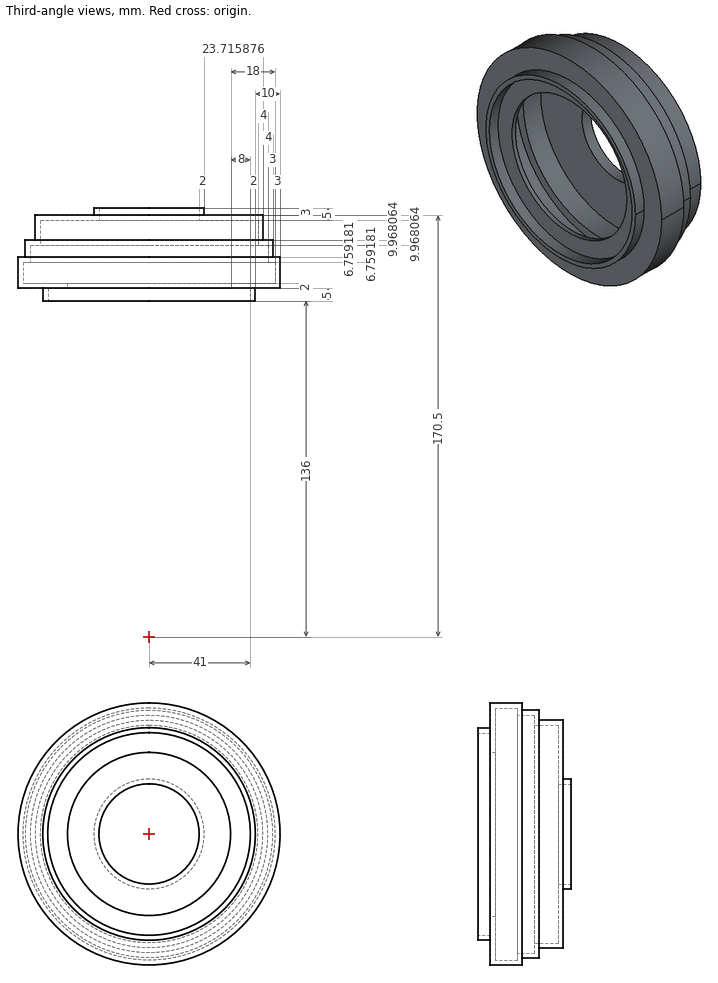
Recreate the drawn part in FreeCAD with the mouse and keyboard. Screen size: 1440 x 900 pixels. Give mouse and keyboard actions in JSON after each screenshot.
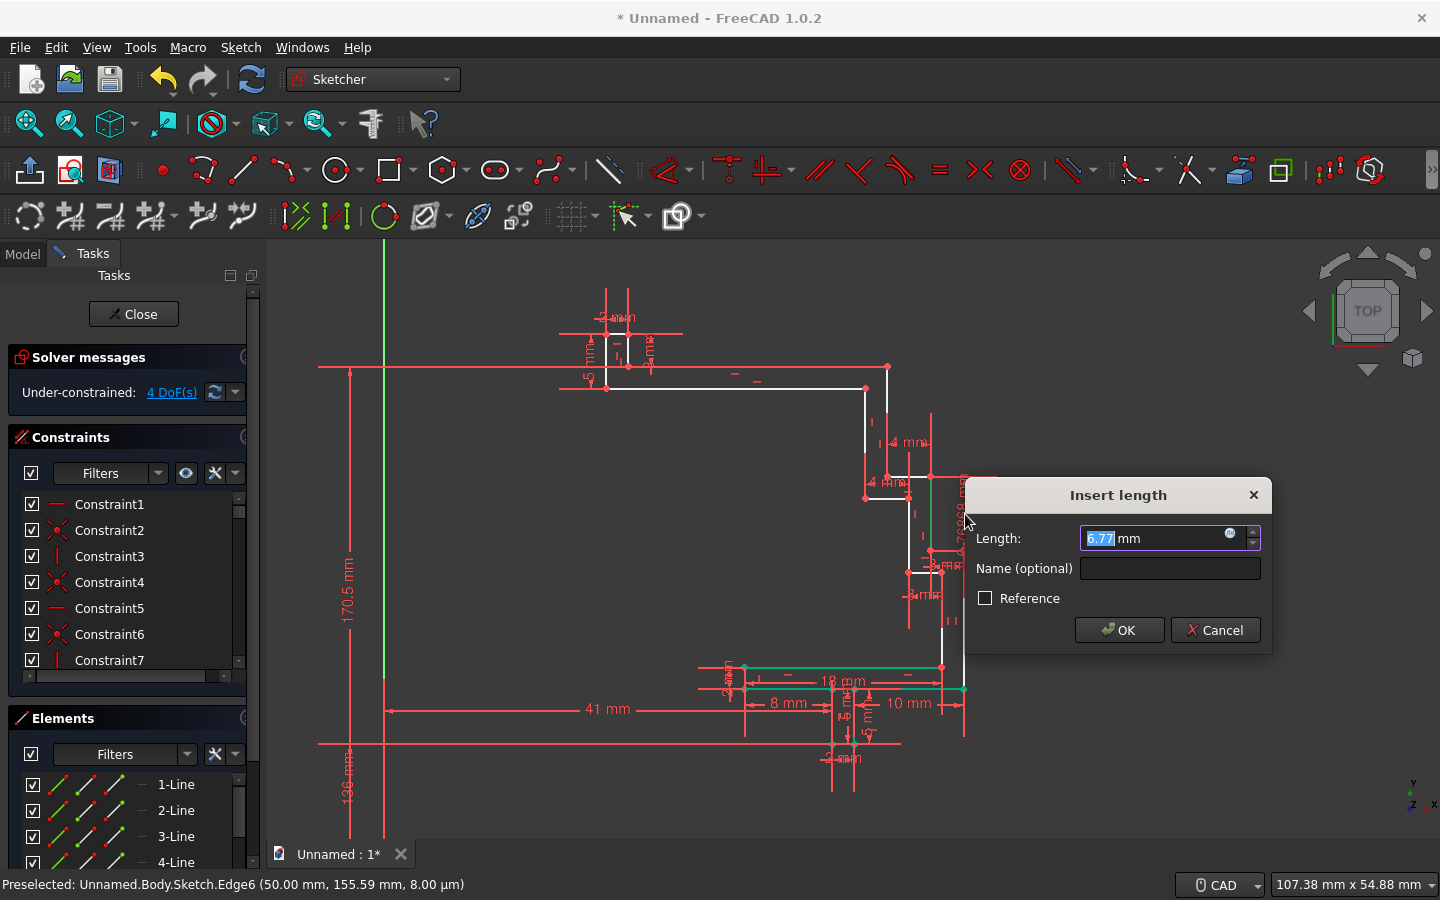
{"action": "type", "text": "6.759181"}
{"action": "key", "text": "Return"}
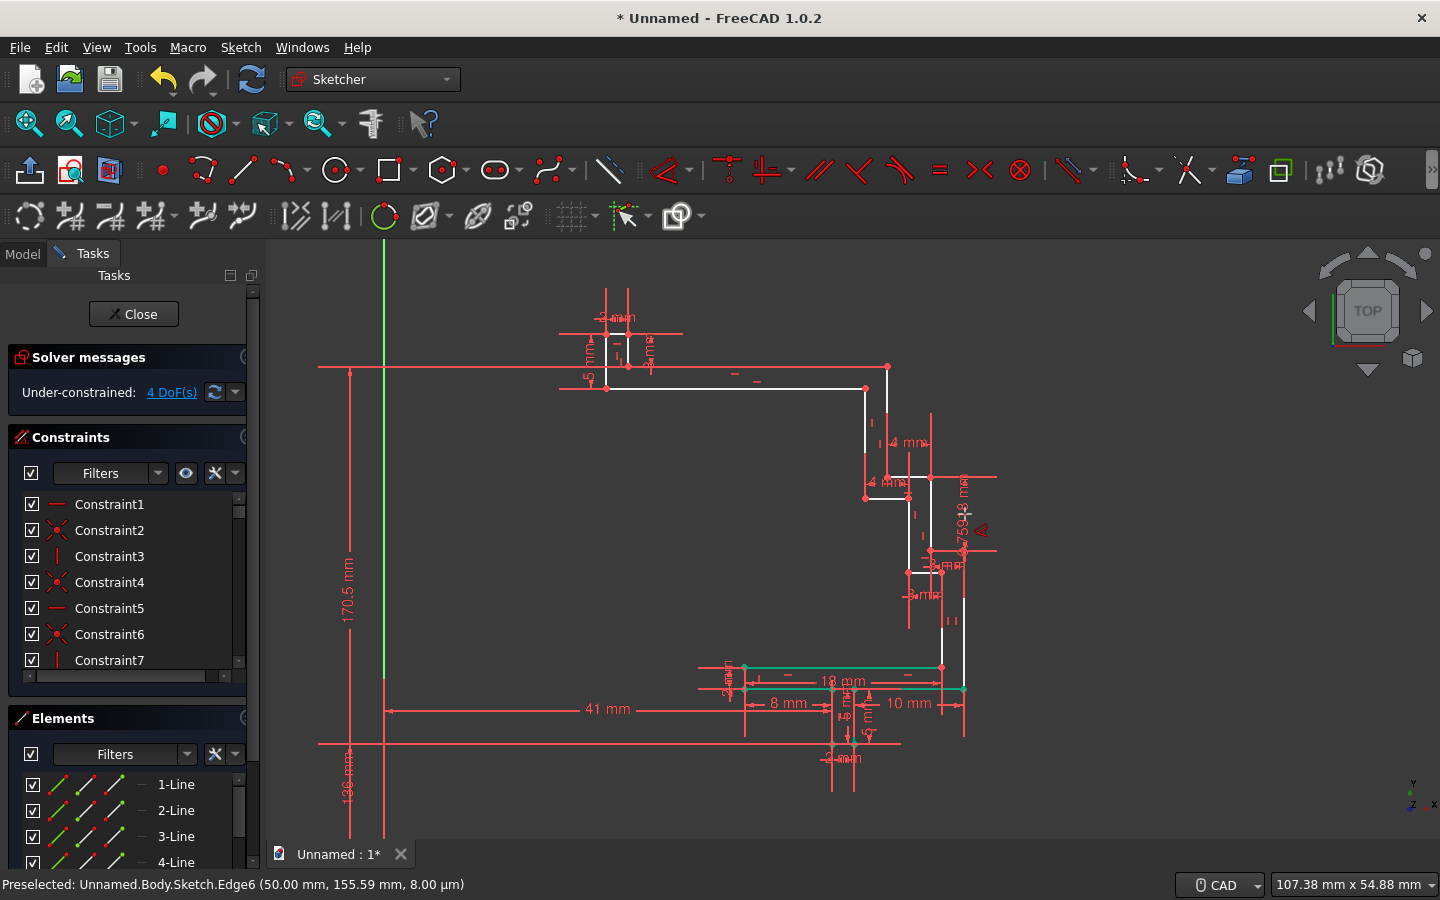
{"action": "left_click", "coordinate": [887, 444]}
{"action": "left_click", "coordinate": [921, 422]}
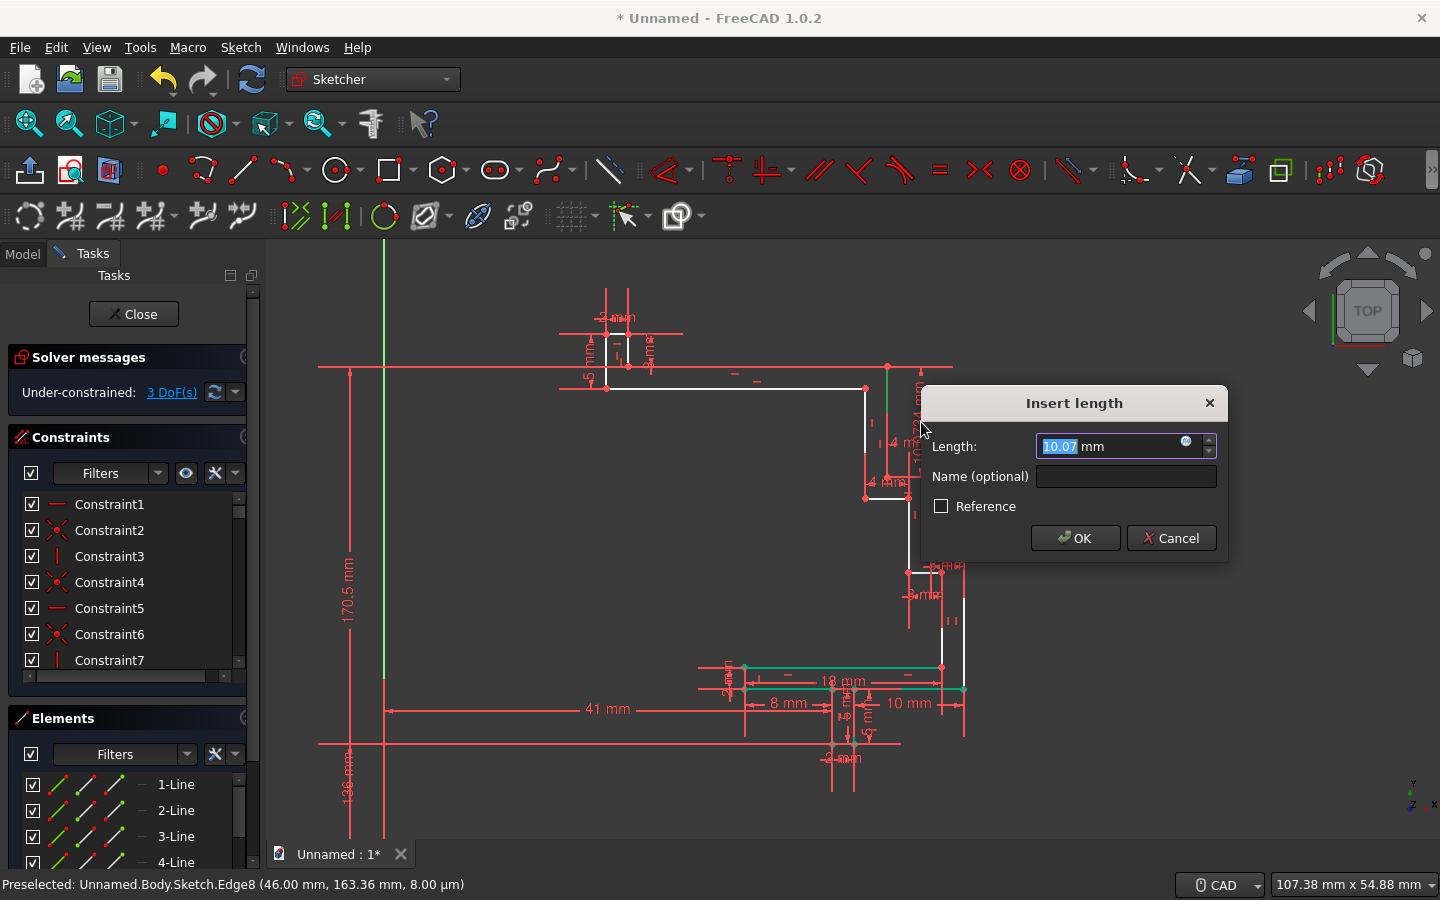
{"action": "type", "text": "9.968064"}
{"action": "key", "text": "Return"}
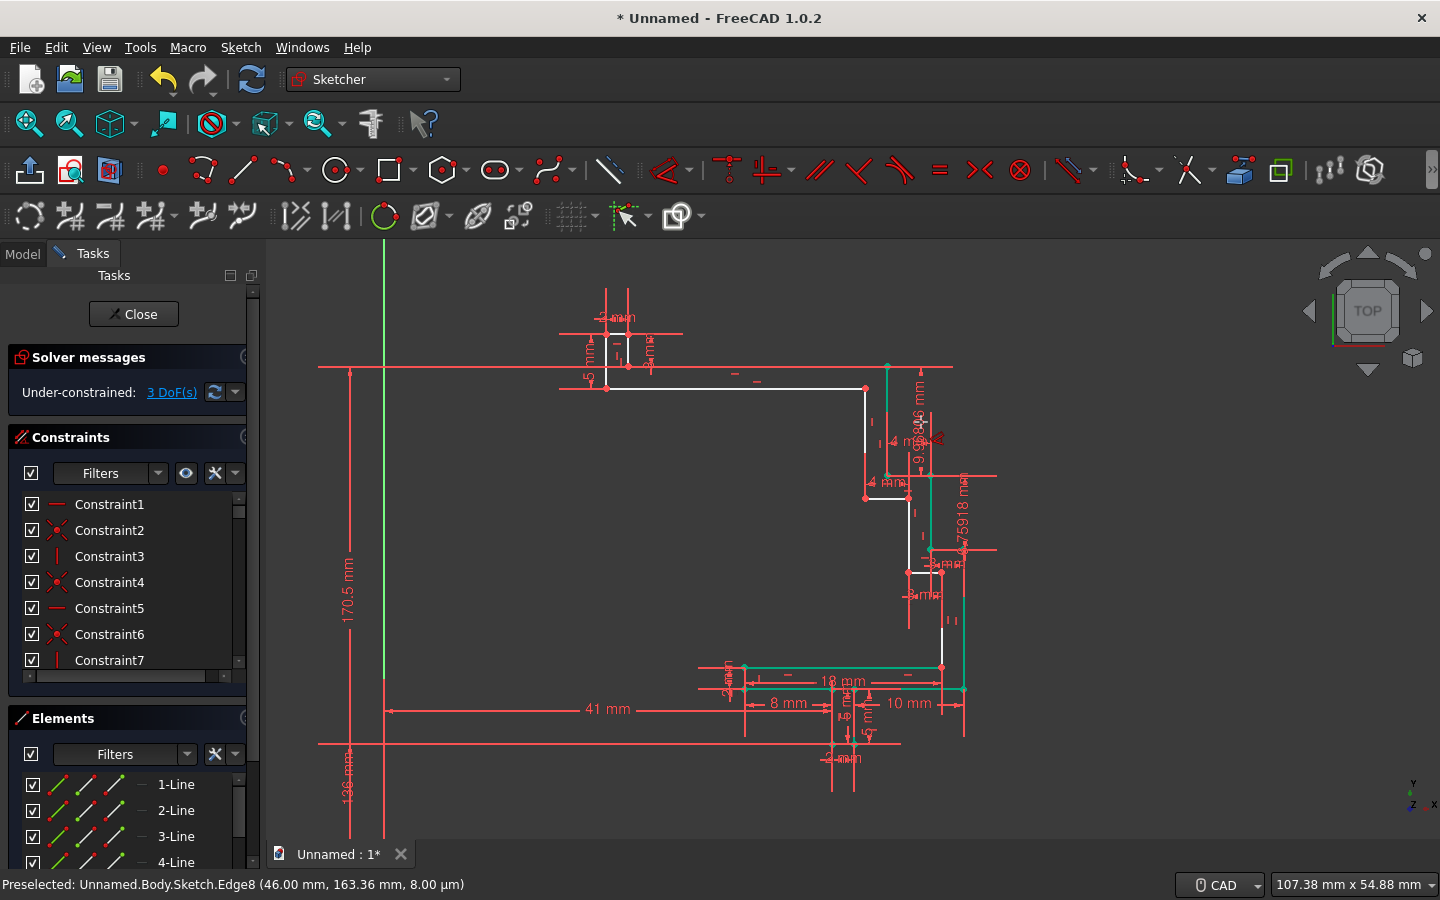
{"action": "left_click", "coordinate": [865, 422]}
{"action": "left_click", "coordinate": [831, 444]}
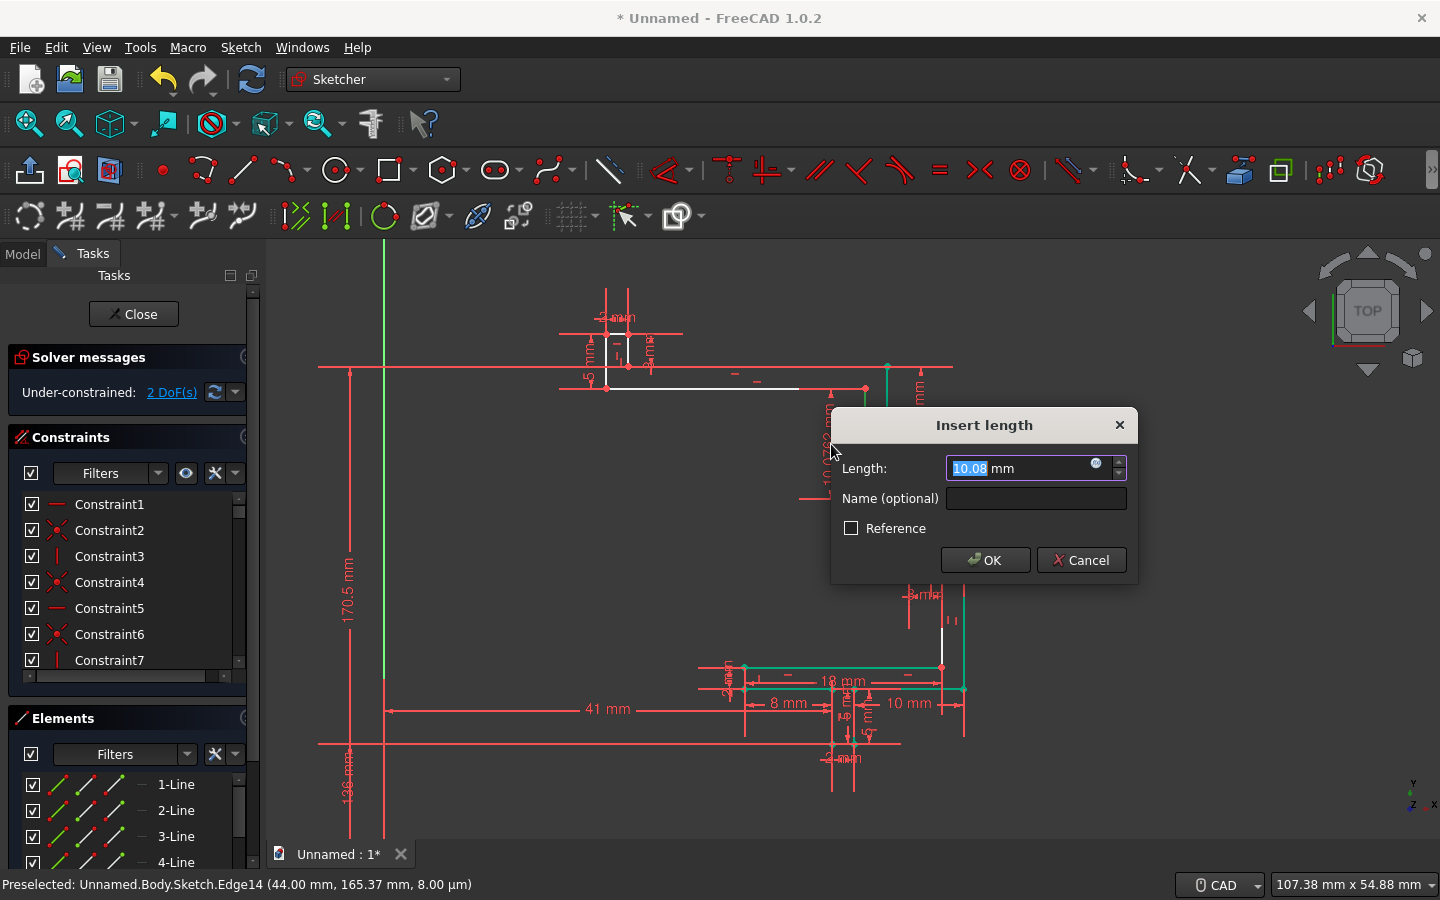
{"action": "type", "text": "9.968064"}
{"action": "key", "text": "Return"}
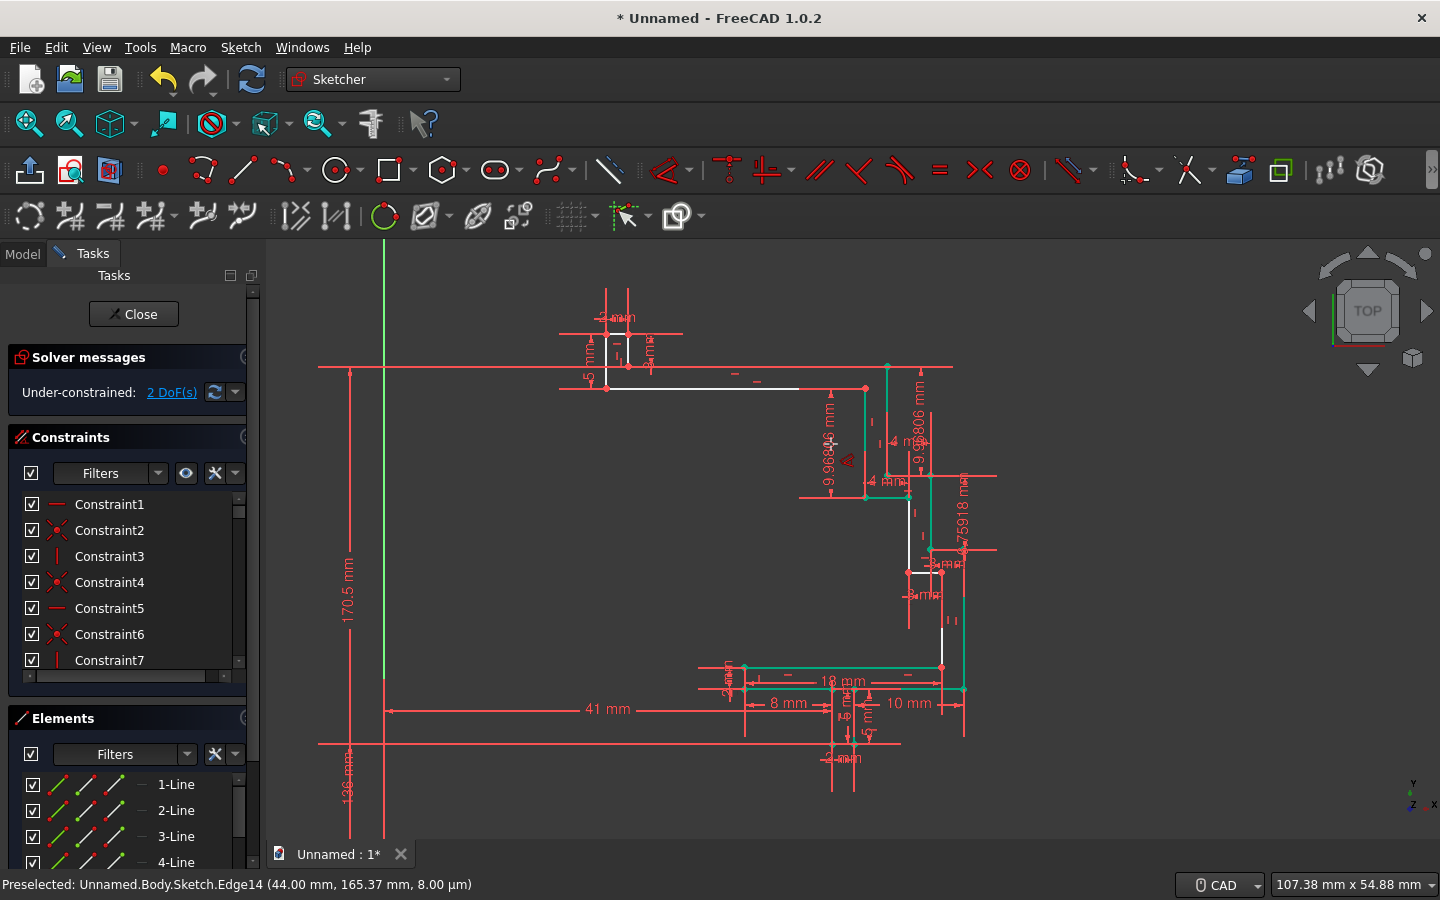
{"action": "left_click", "coordinate": [909, 520]}
{"action": "left_click", "coordinate": [875, 535]}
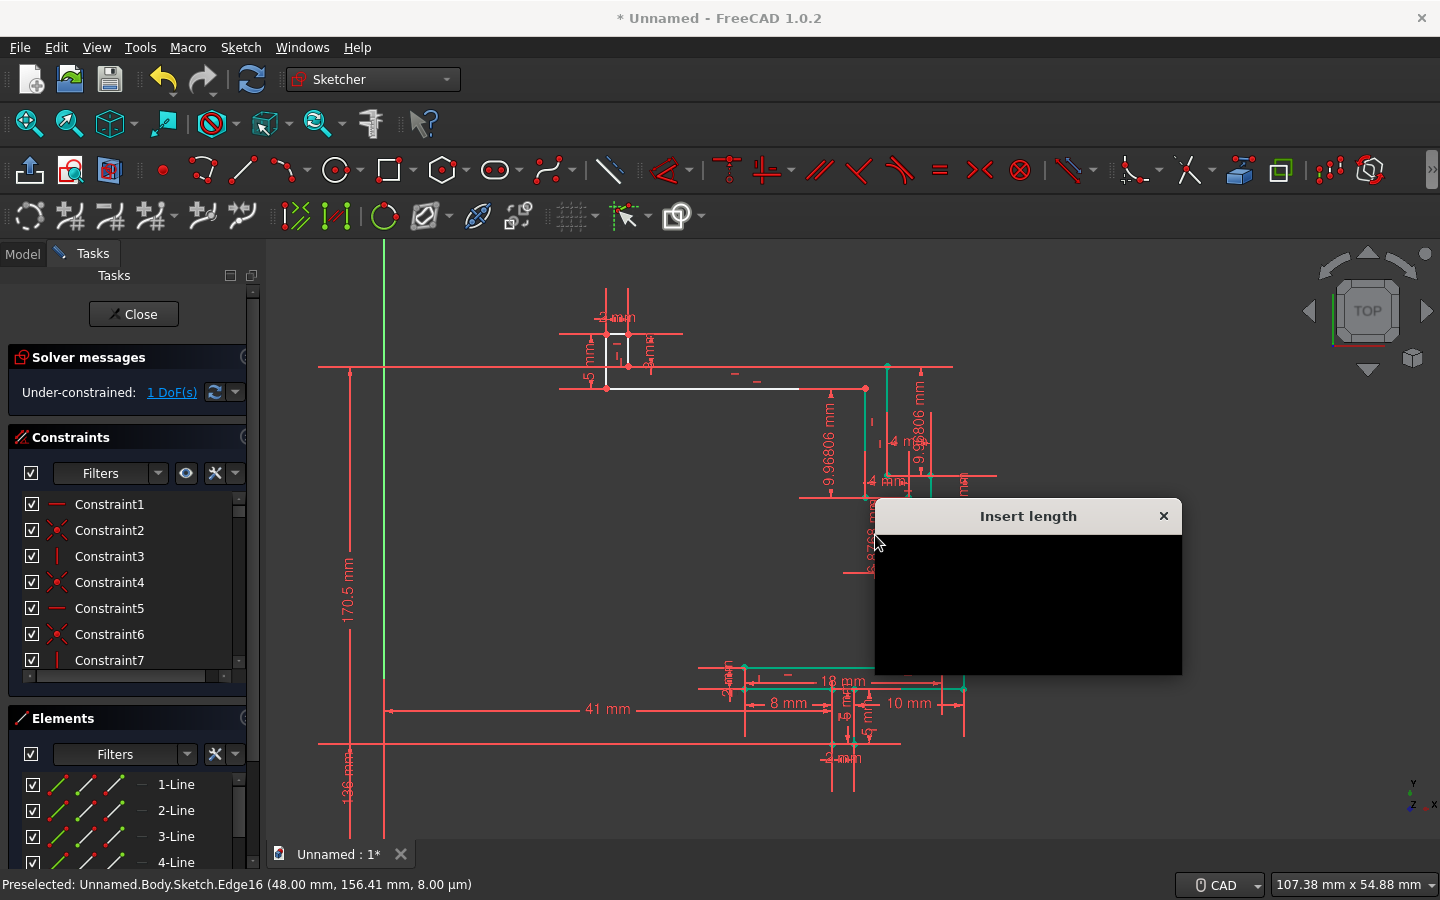
{"action": "type", "text": "6.759181"}
{"action": "key", "text": "Return"}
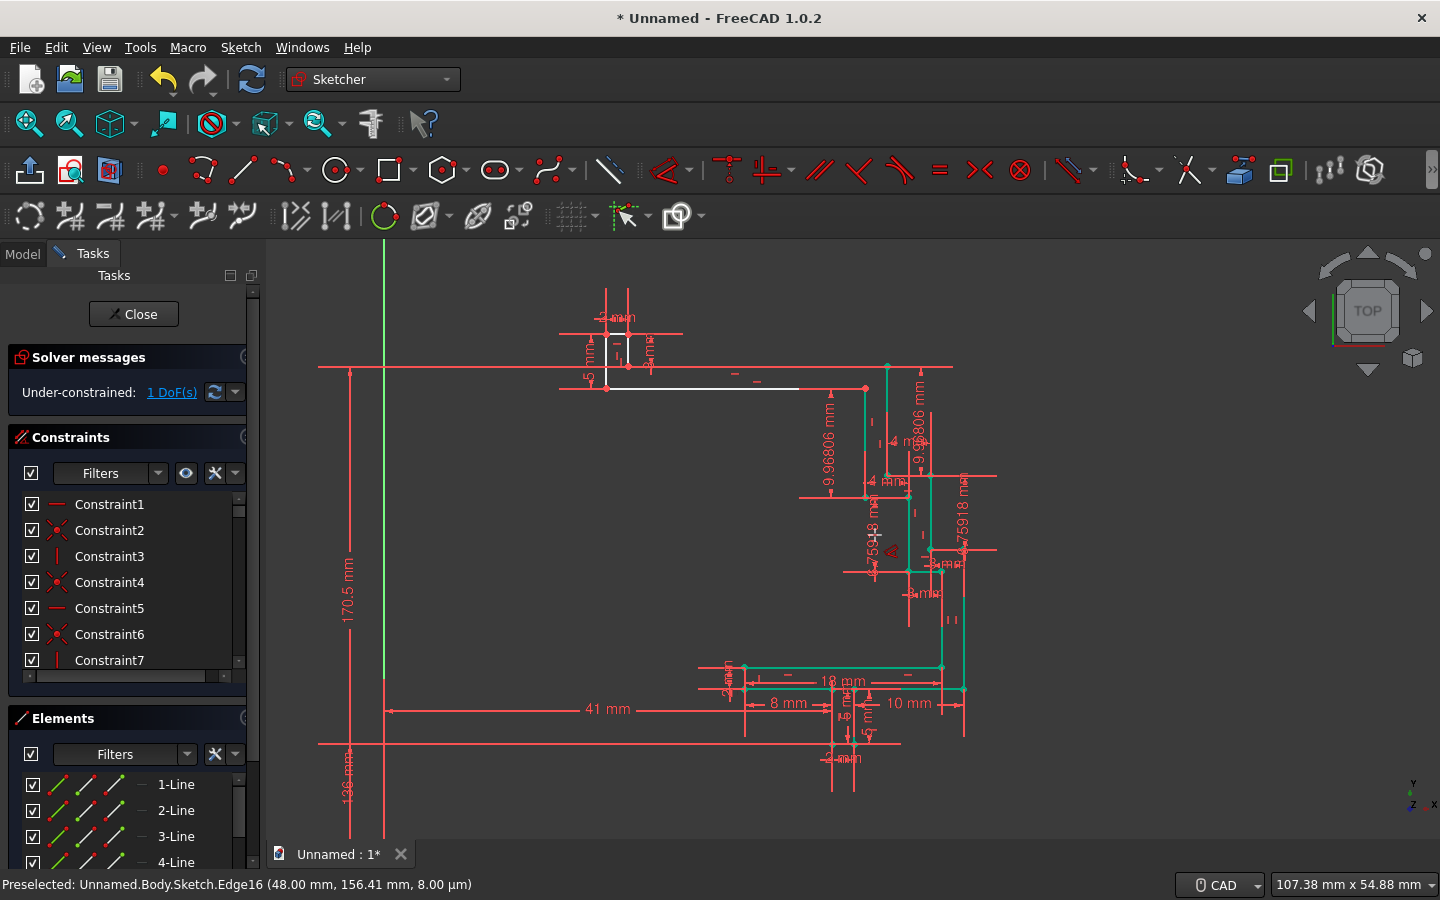
{"action": "left_click", "coordinate": [809, 367]}
{"action": "left_click", "coordinate": [758, 333]}